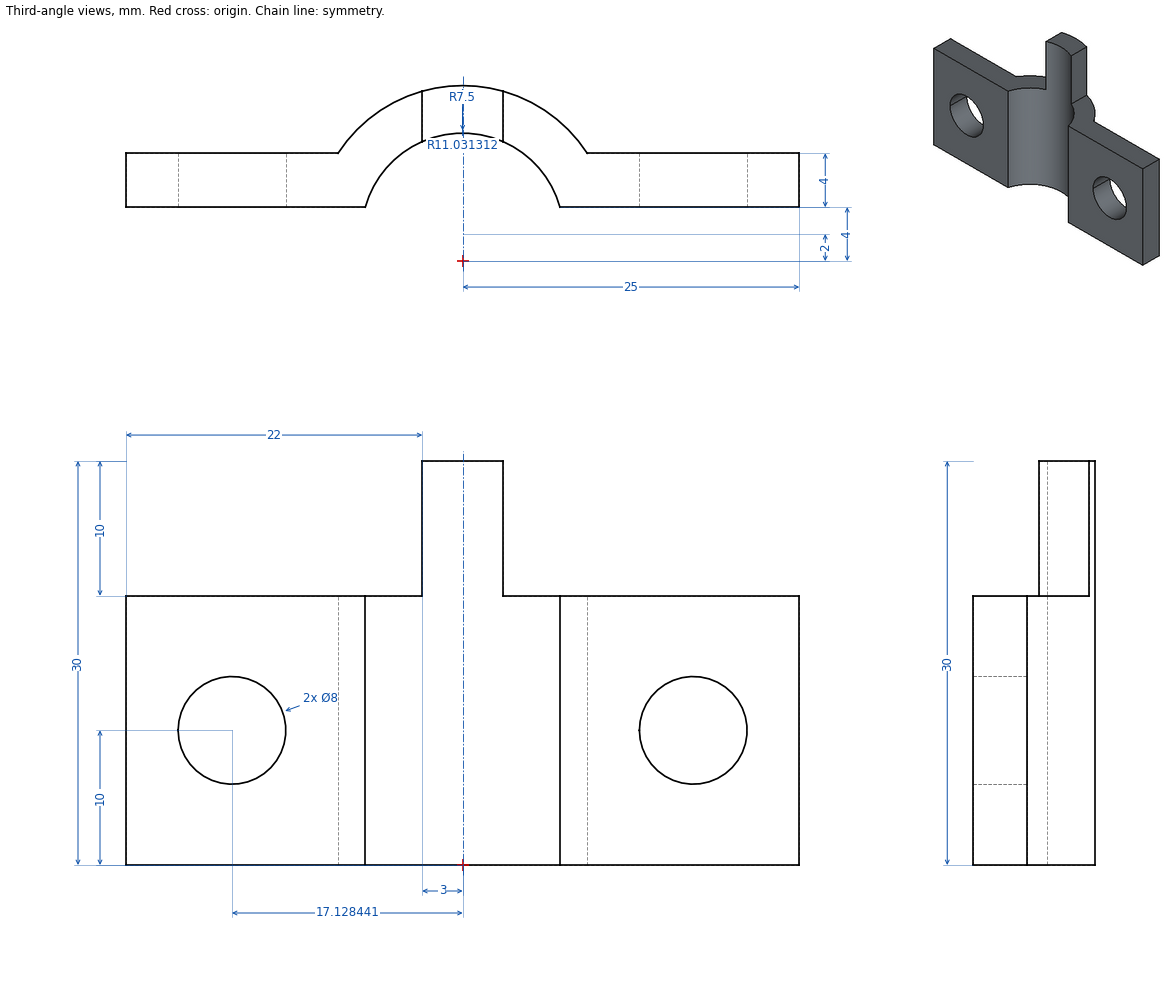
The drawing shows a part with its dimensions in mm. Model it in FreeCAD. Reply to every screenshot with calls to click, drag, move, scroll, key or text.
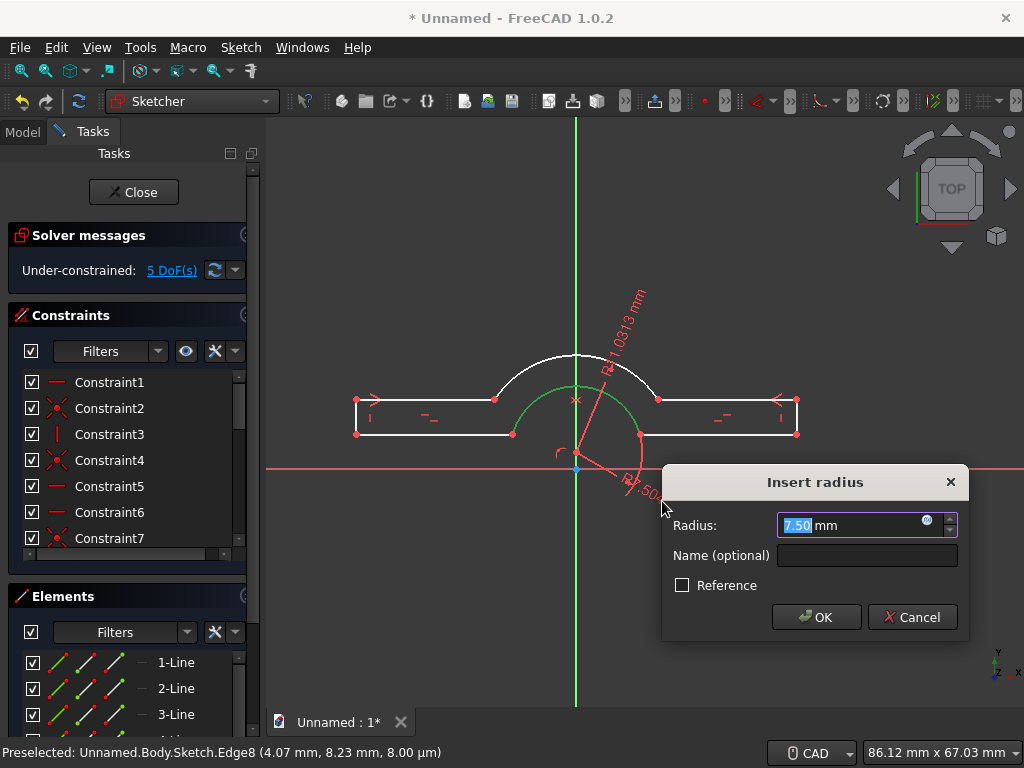
text(7.5)
key(Return)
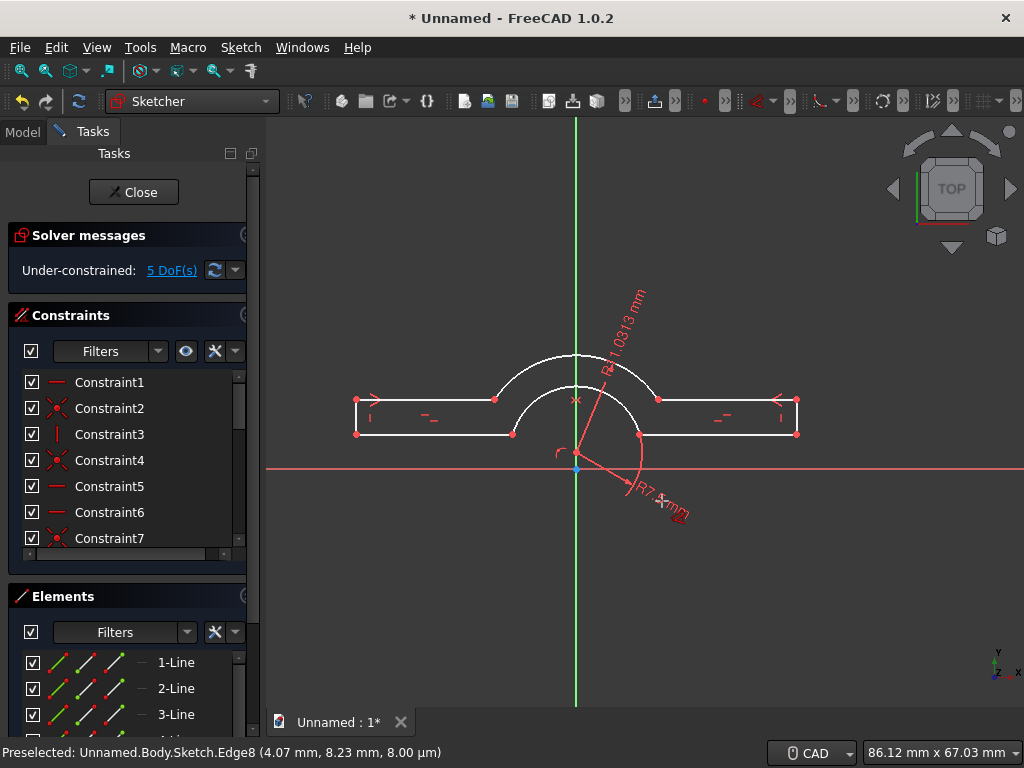
scroll(797, 424, up, 2)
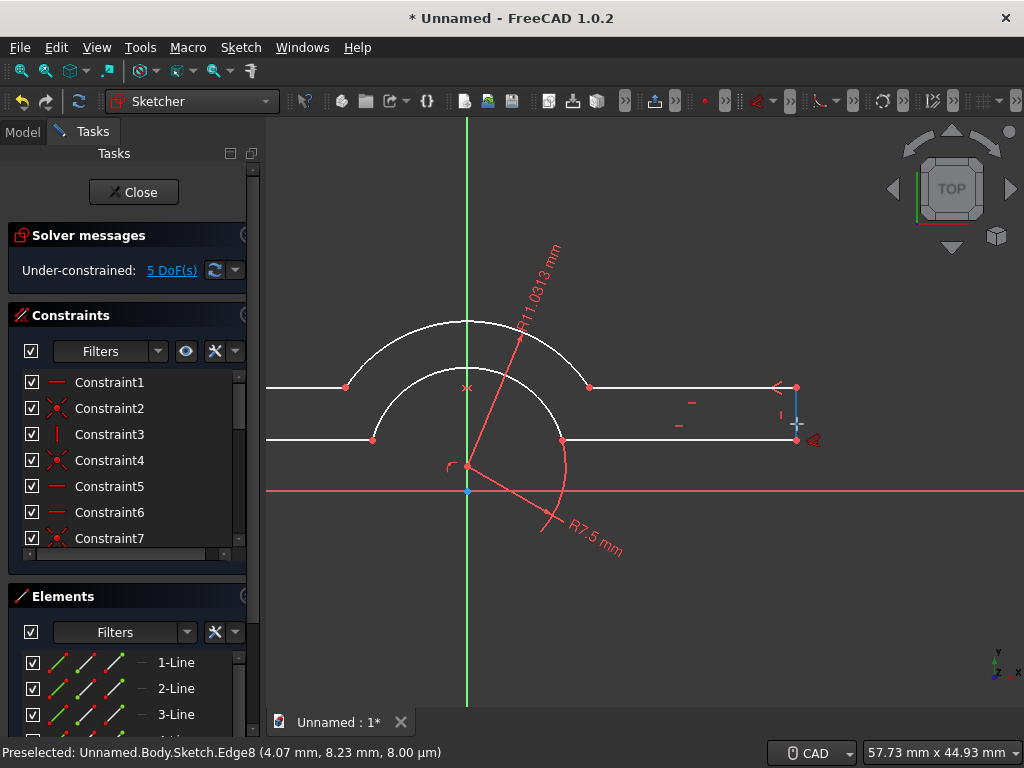
click(796, 424)
click(830, 414)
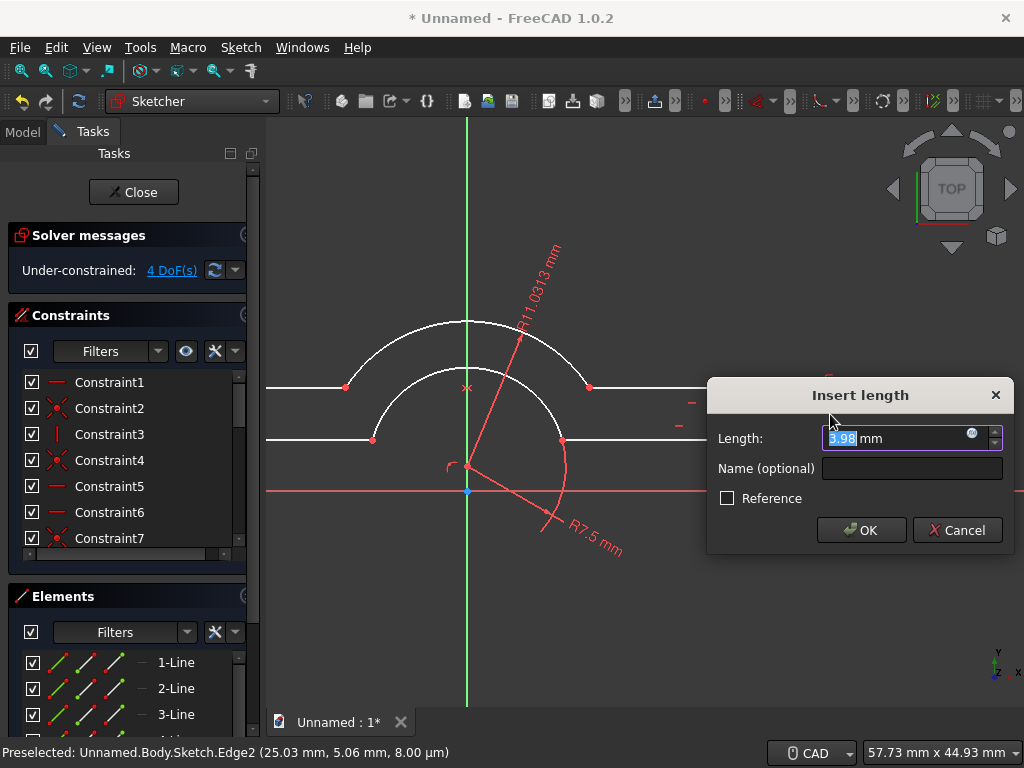
text(4)
key(Return)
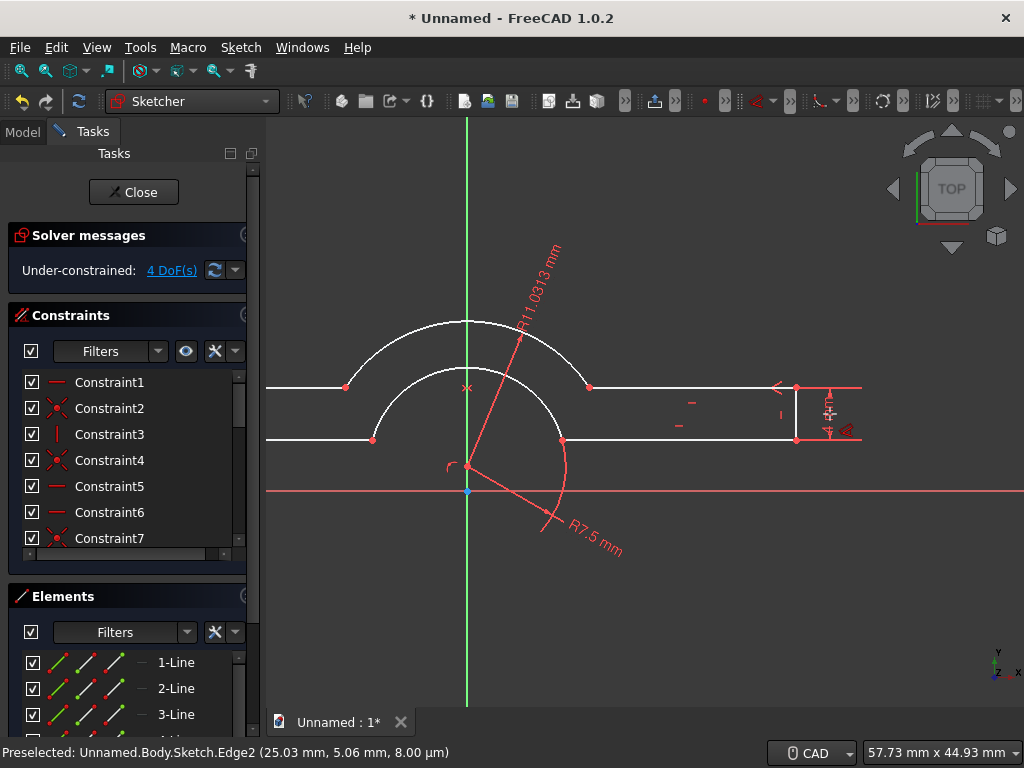
scroll(798, 424, down, 2)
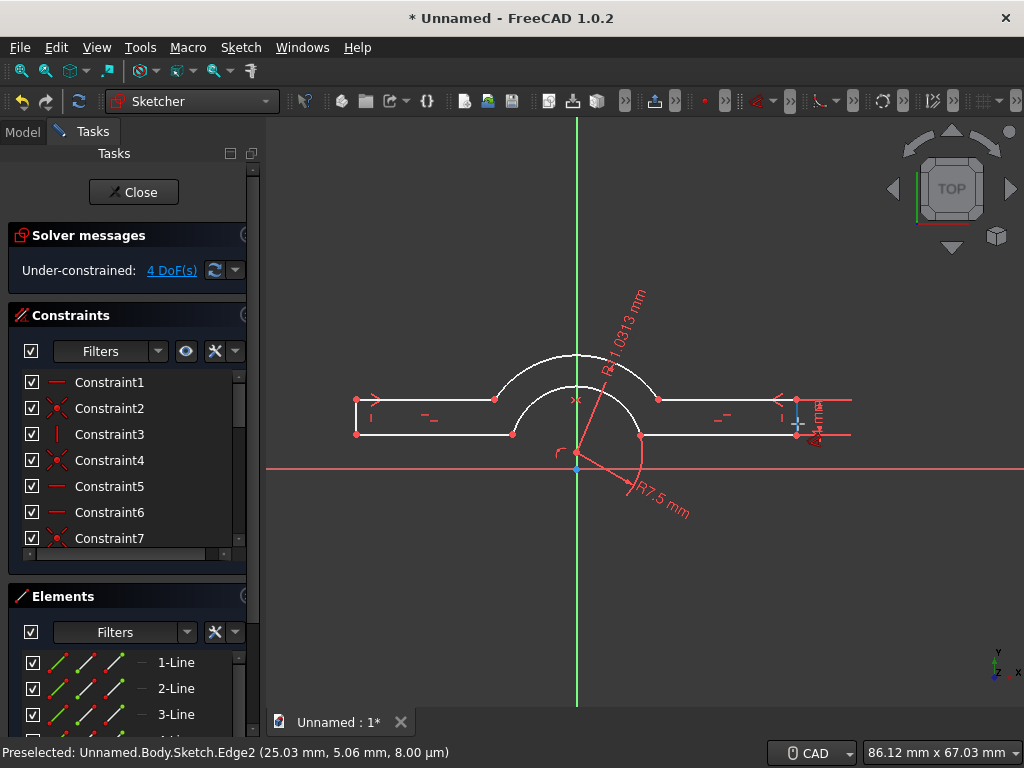
scroll(356, 410, up, 2)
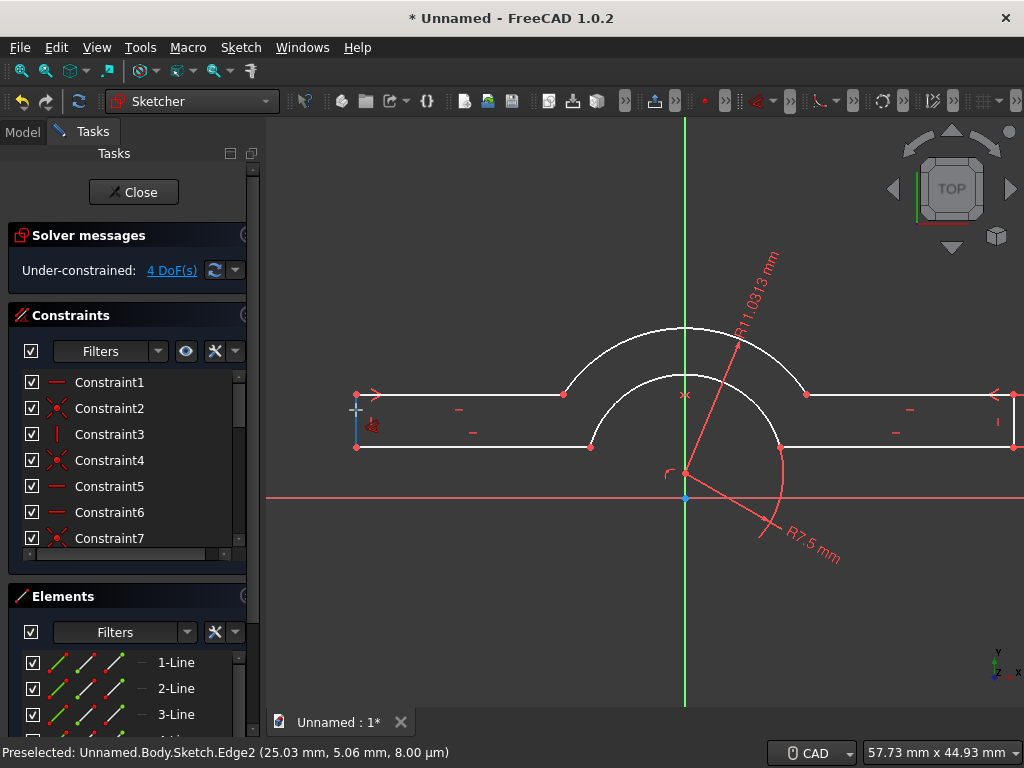
click(356, 411)
click(322, 421)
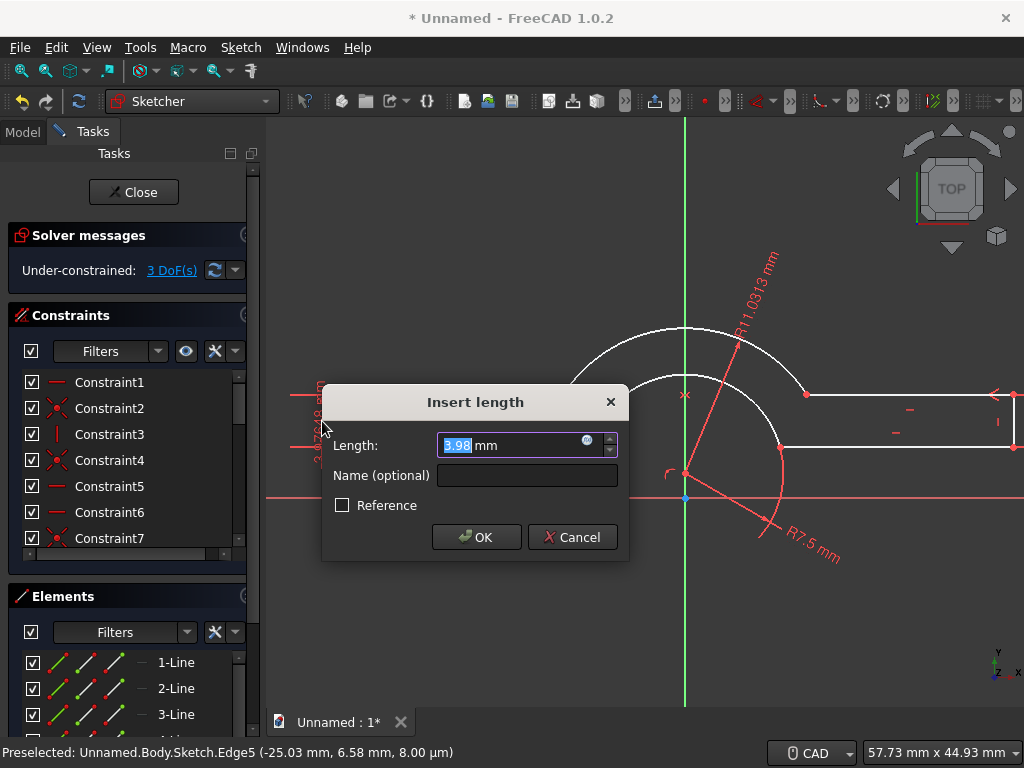
text(4)
key(Return)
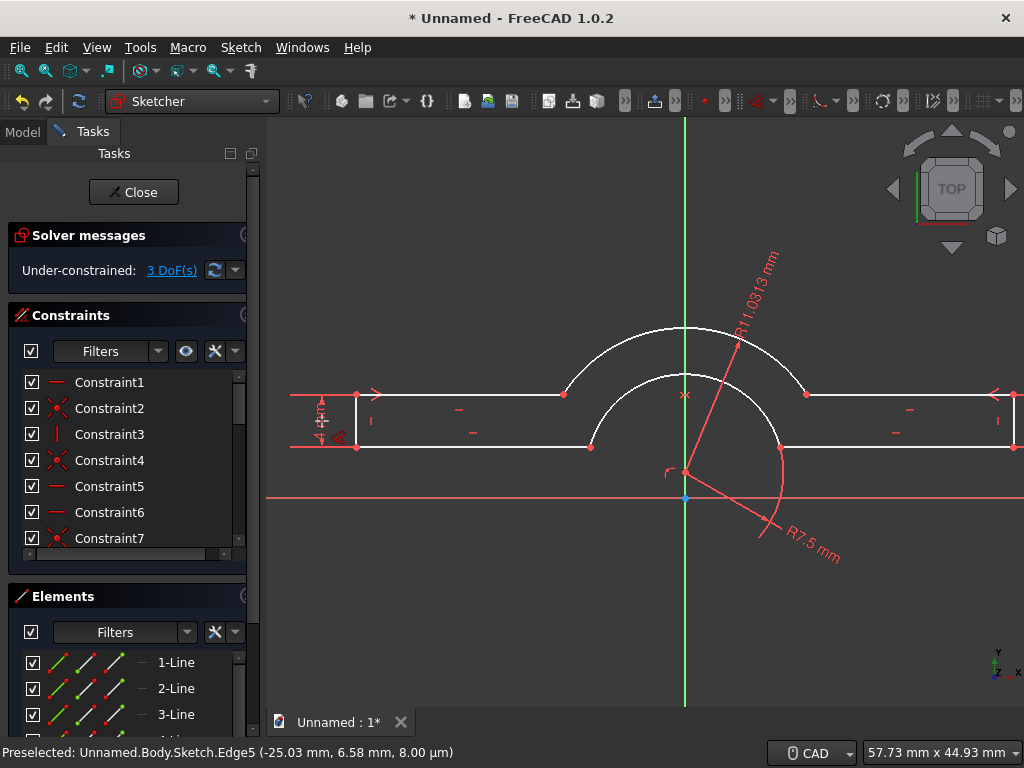
click(780, 447)
click(814, 473)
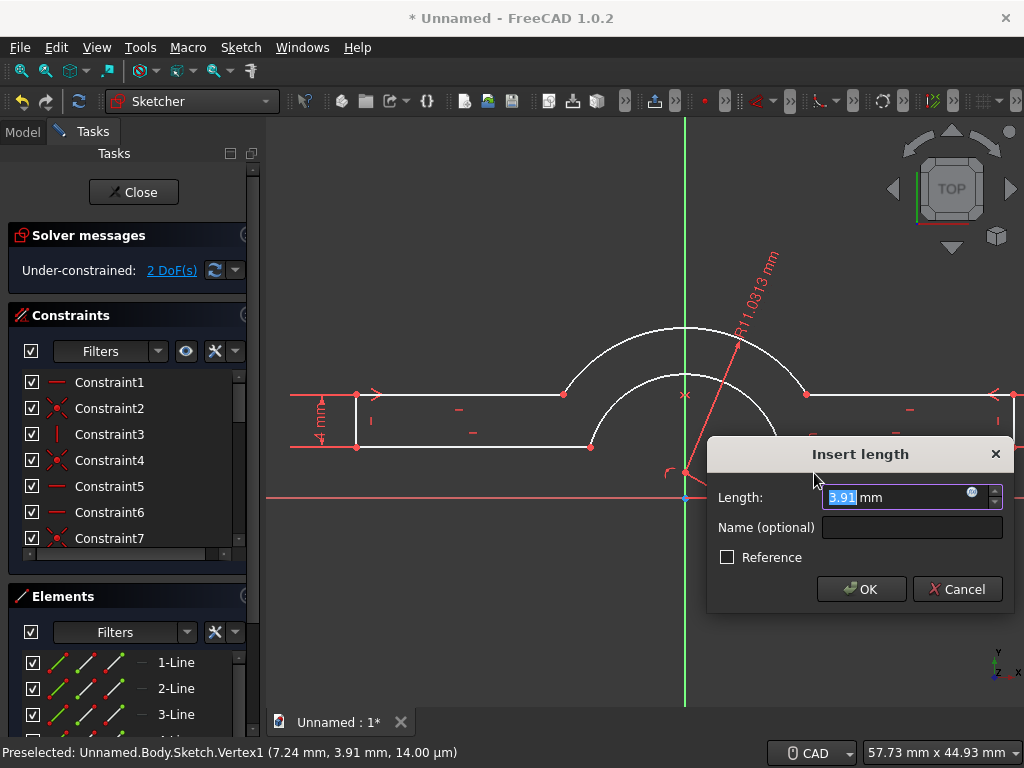
text(4)
key(Return)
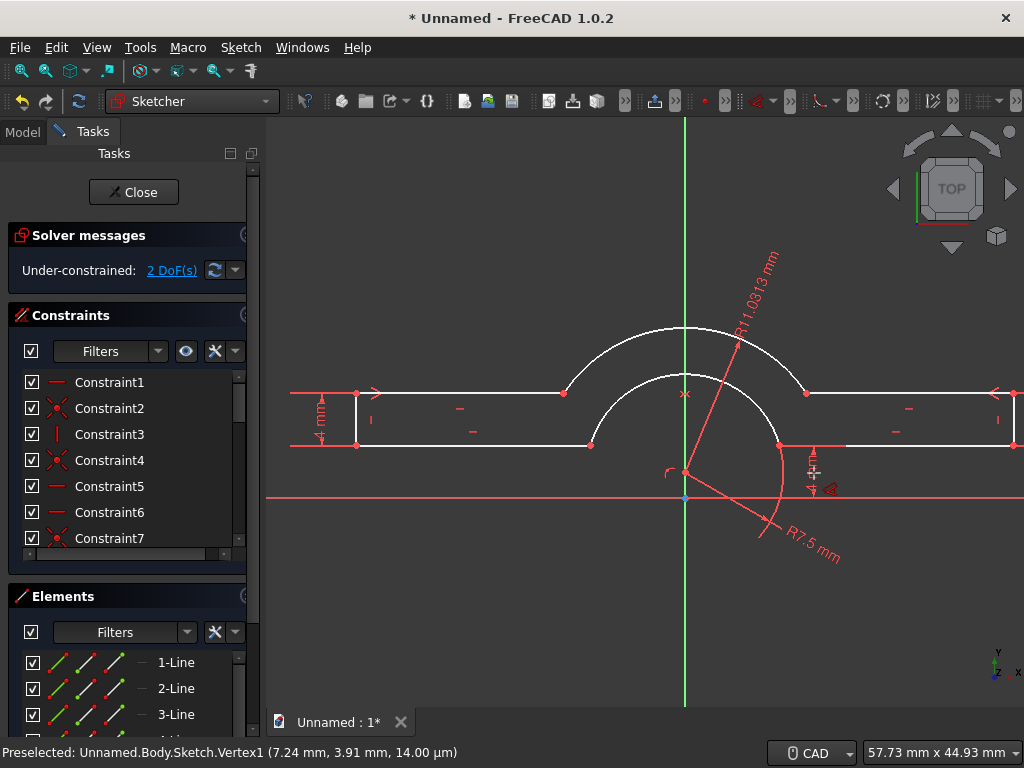
scroll(685, 473, up, 3)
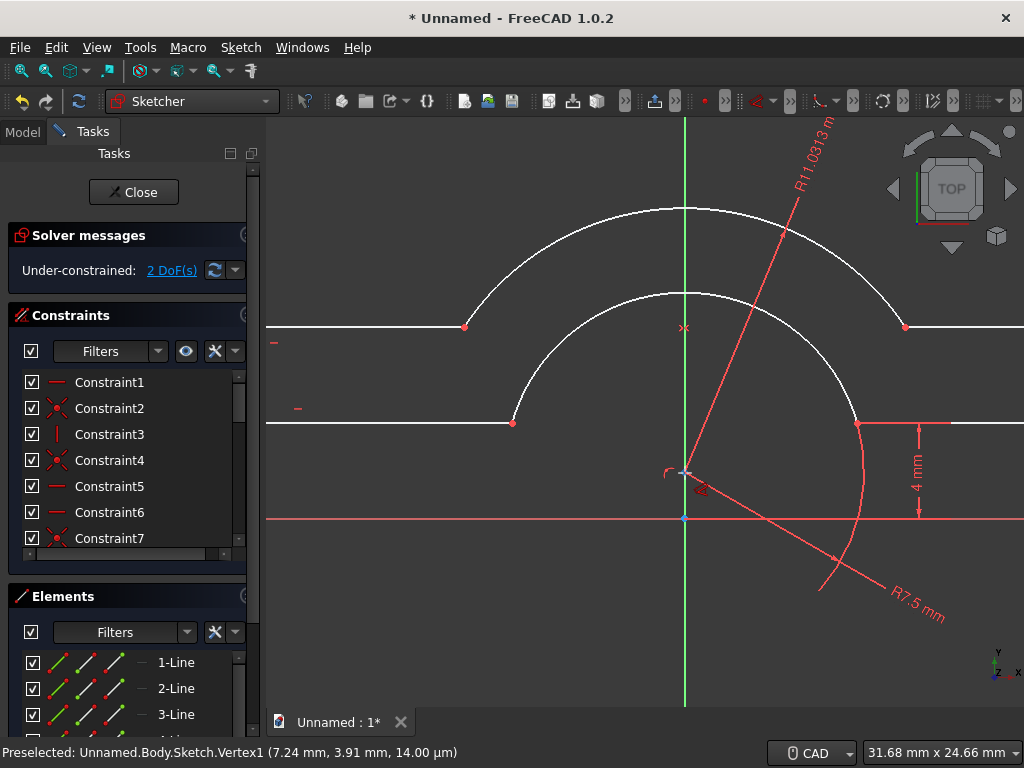
click(685, 472)
click(719, 495)